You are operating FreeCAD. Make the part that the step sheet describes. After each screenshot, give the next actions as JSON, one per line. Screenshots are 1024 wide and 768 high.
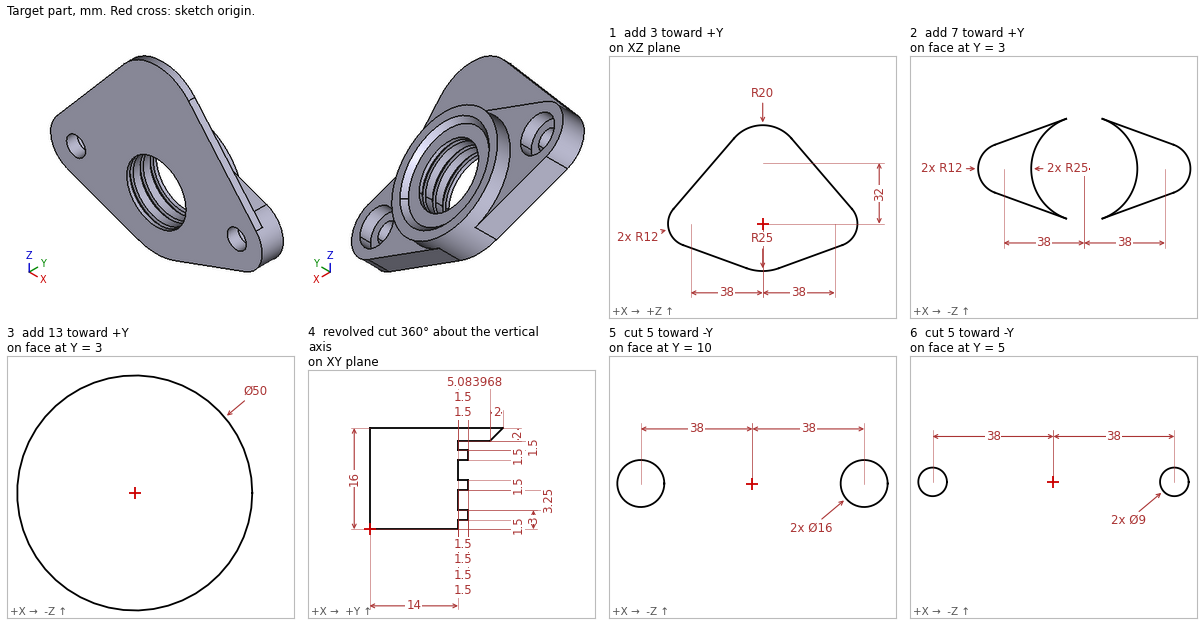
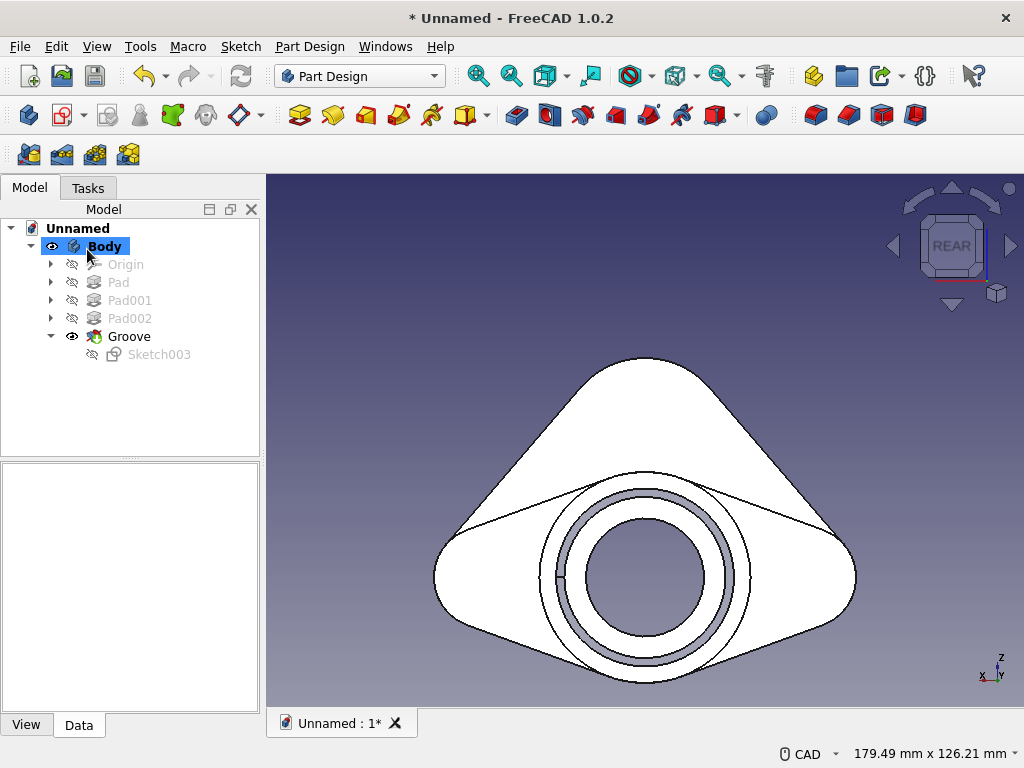
{"action": "left_click", "coordinate": [496, 576]}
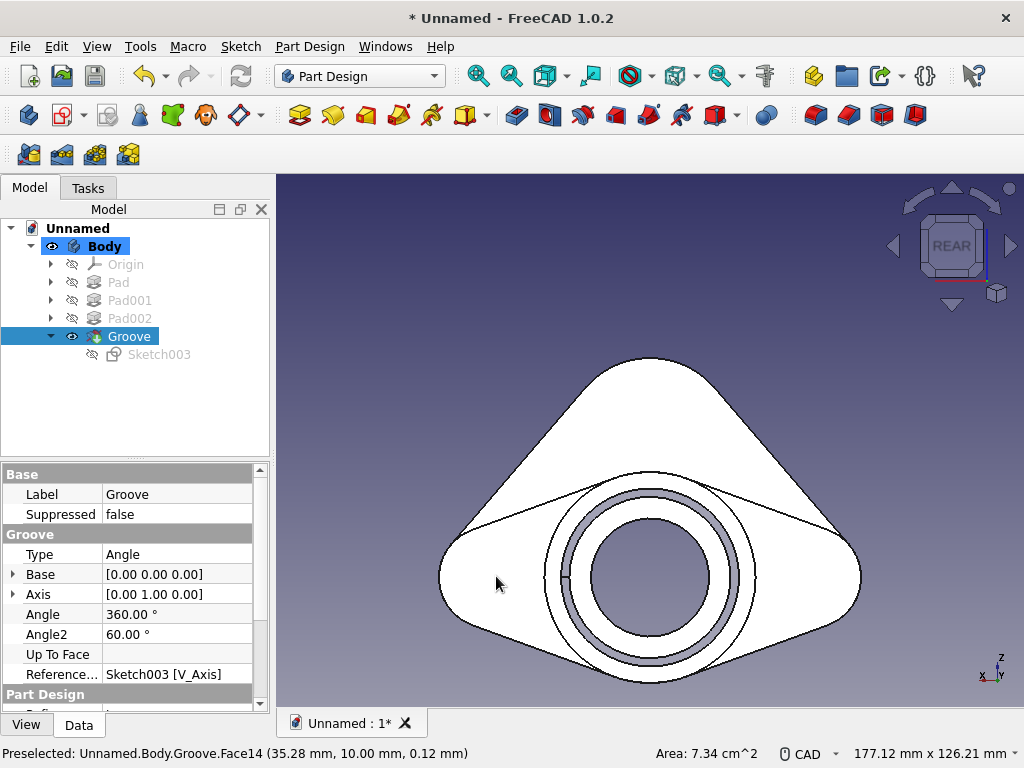
{"action": "left_click", "coordinate": [62, 116]}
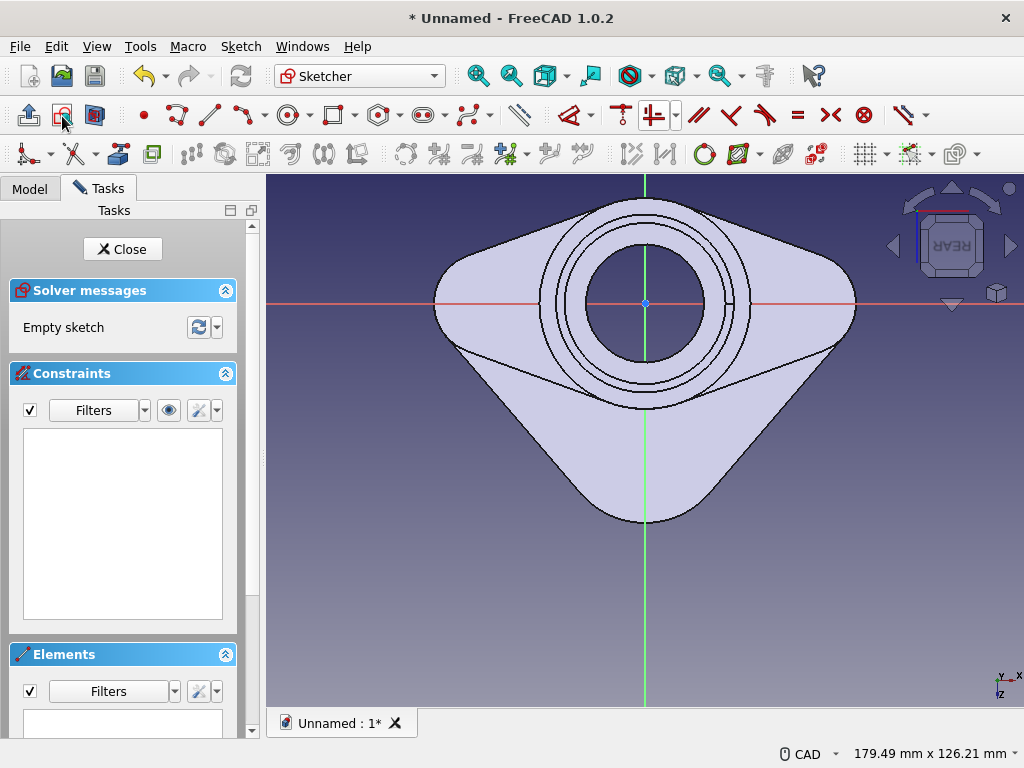
{"action": "left_click", "coordinate": [95, 116]}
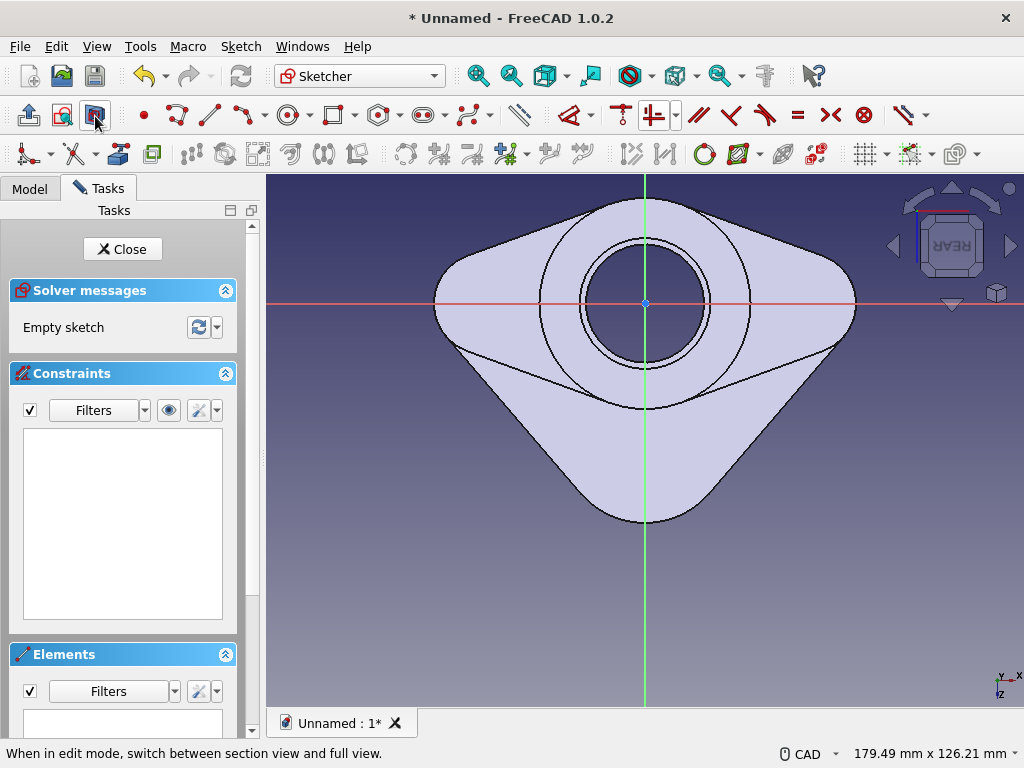
{"action": "scroll", "coordinate": [294, 679], "scroll_direction": "down", "scroll_amount": 1}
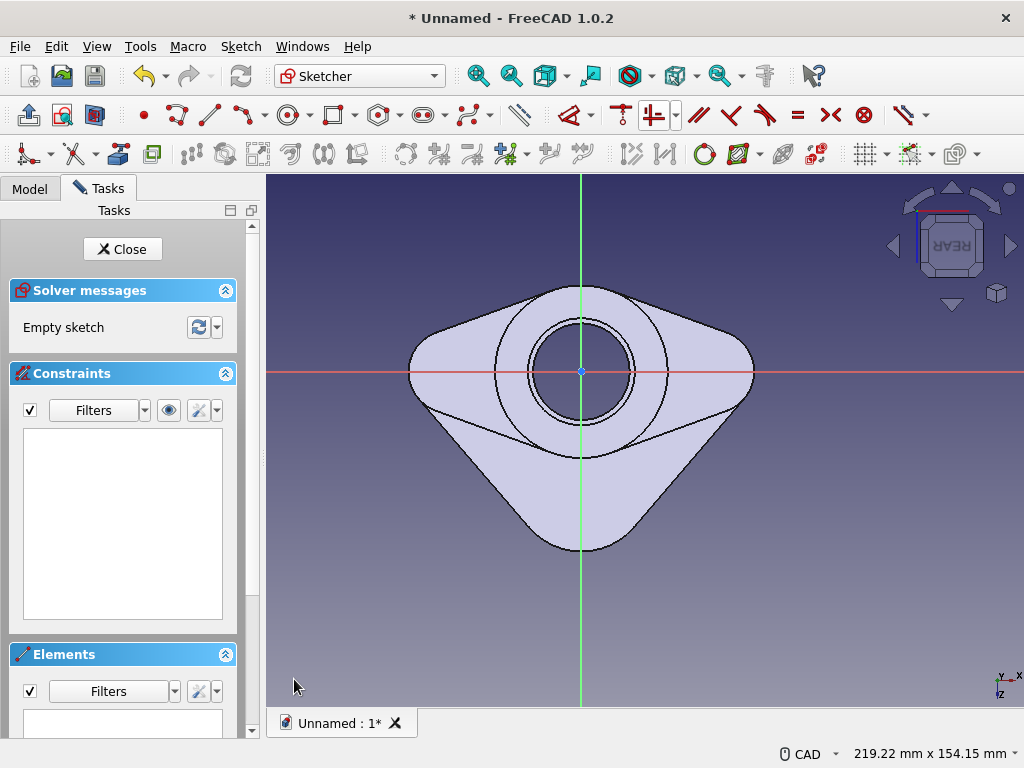
{"action": "left_click", "coordinate": [288, 116]}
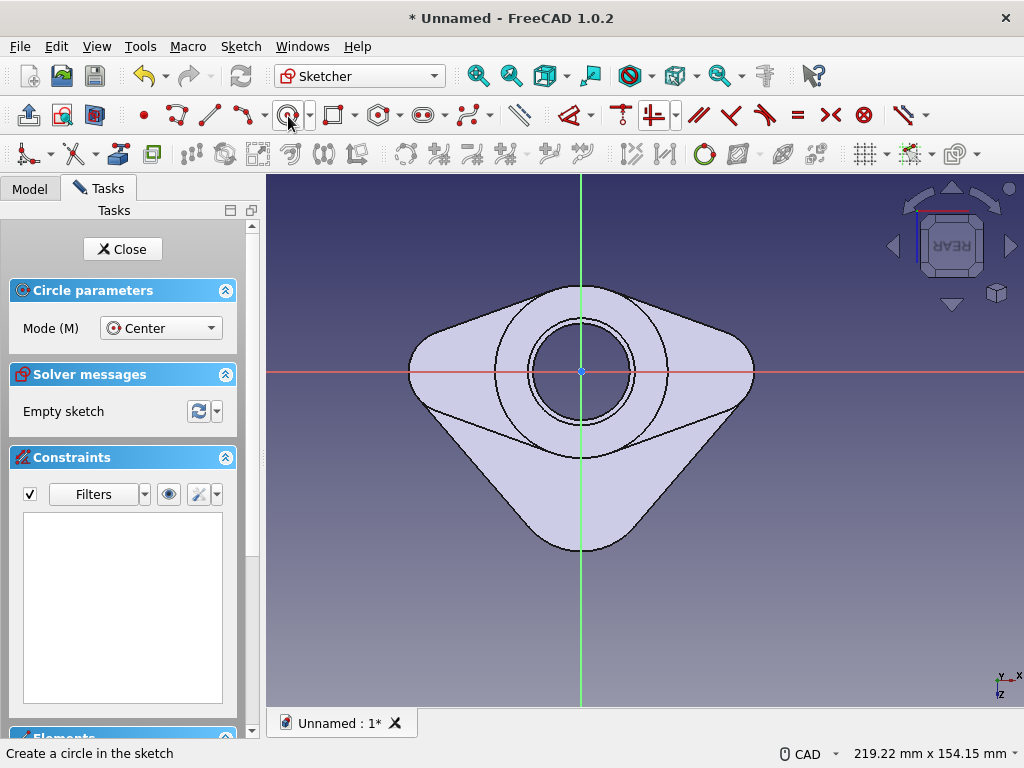
{"action": "left_click", "coordinate": [713, 372]}
{"action": "left_click", "coordinate": [732, 352]}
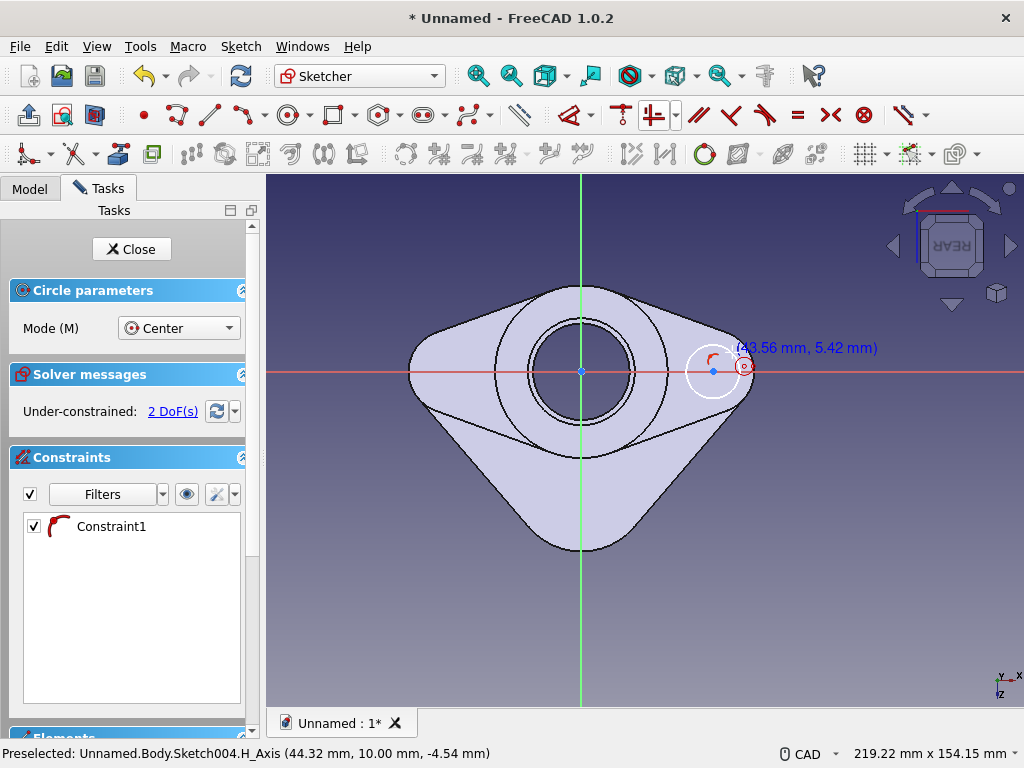
{"action": "left_click", "coordinate": [450, 372]}
{"action": "left_click", "coordinate": [470, 352]}
{"action": "key", "text": "Escape"}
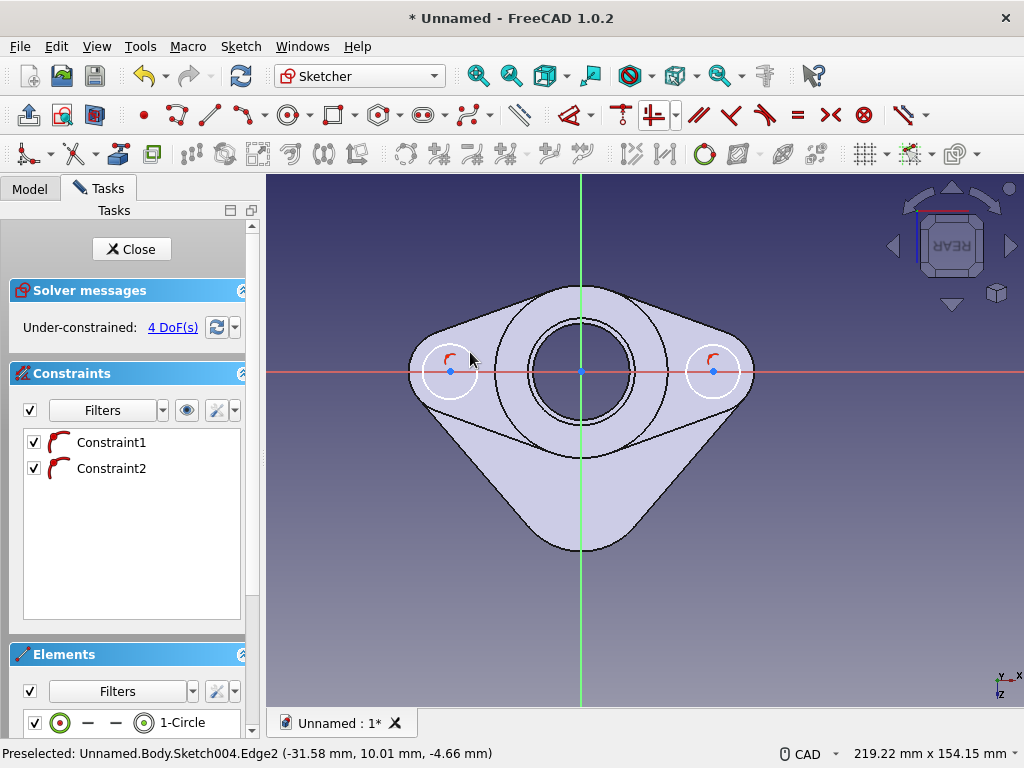
{"action": "left_click", "coordinate": [732, 353]}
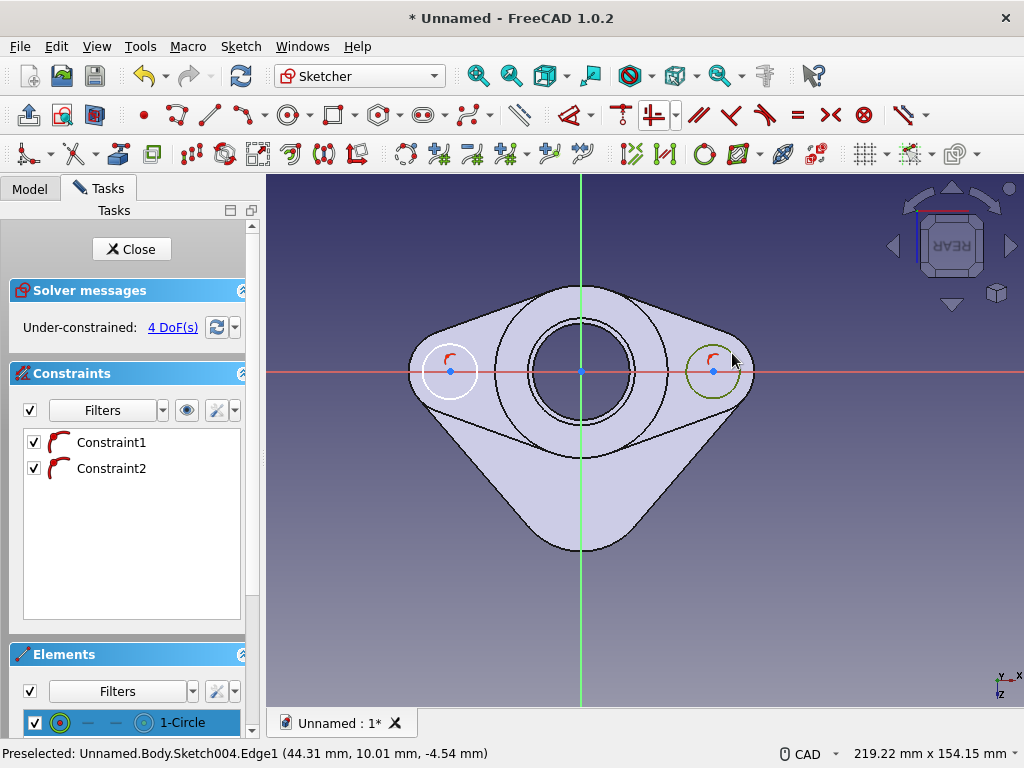
{"action": "left_click", "coordinate": [469, 352]}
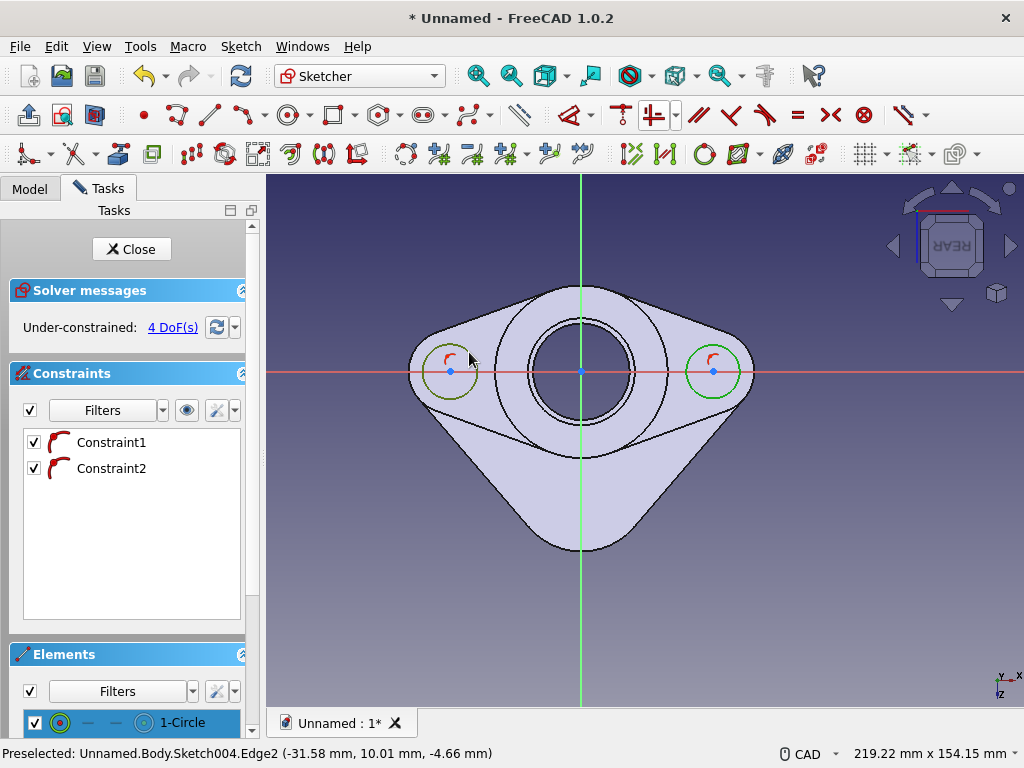
{"action": "left_click", "coordinate": [798, 116]}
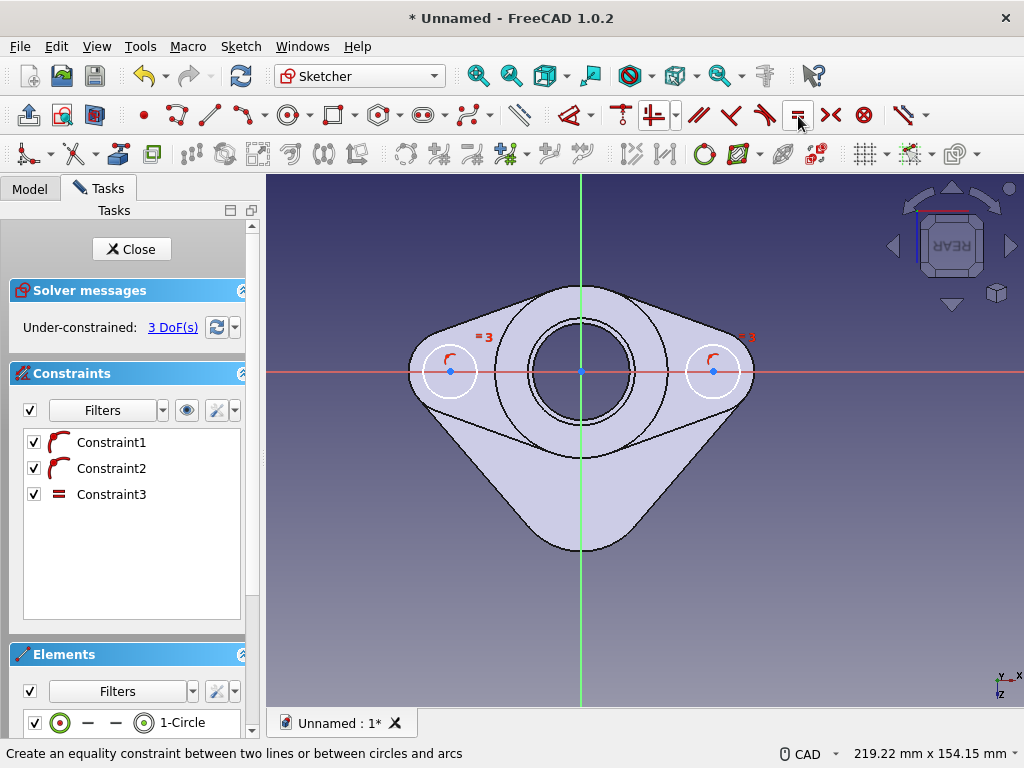
{"action": "left_click", "coordinate": [568, 116]}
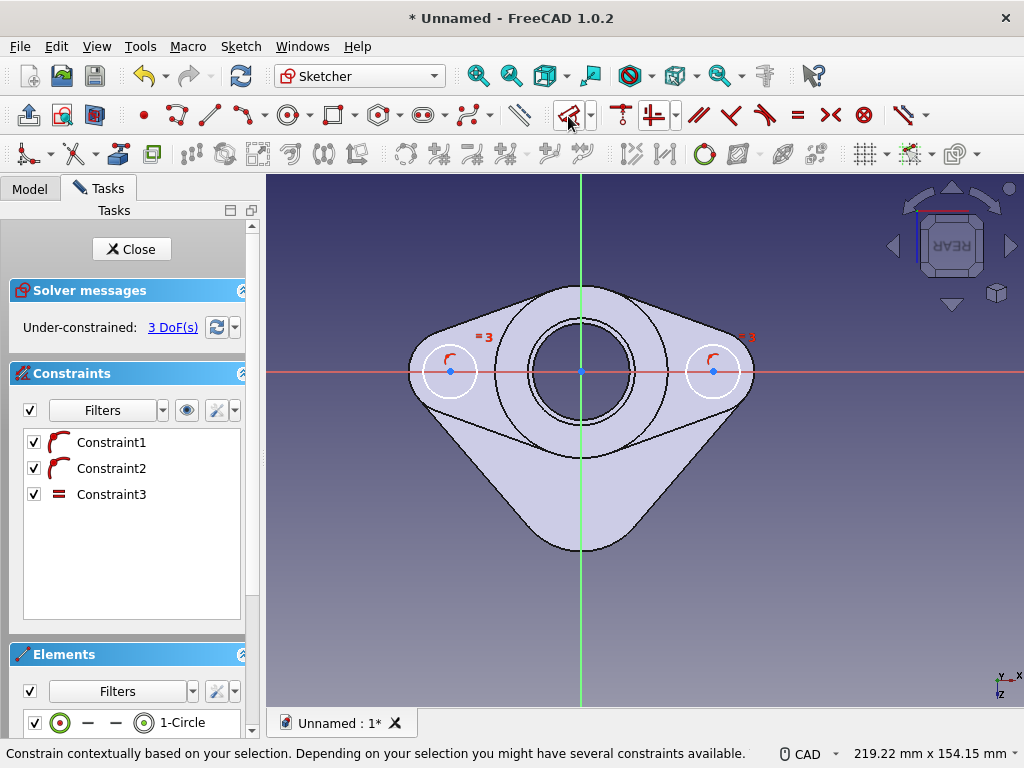
{"action": "left_click", "coordinate": [732, 353]}
{"action": "left_click", "coordinate": [755, 331]}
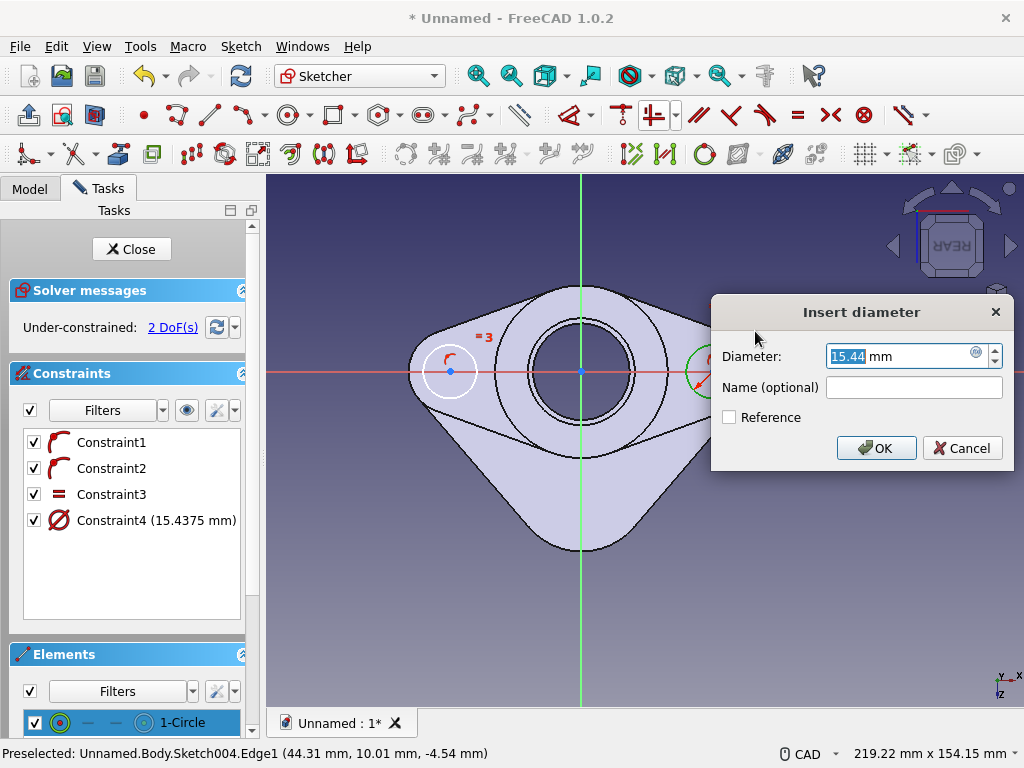
{"action": "type", "text": "16"}
{"action": "key", "text": "Return"}